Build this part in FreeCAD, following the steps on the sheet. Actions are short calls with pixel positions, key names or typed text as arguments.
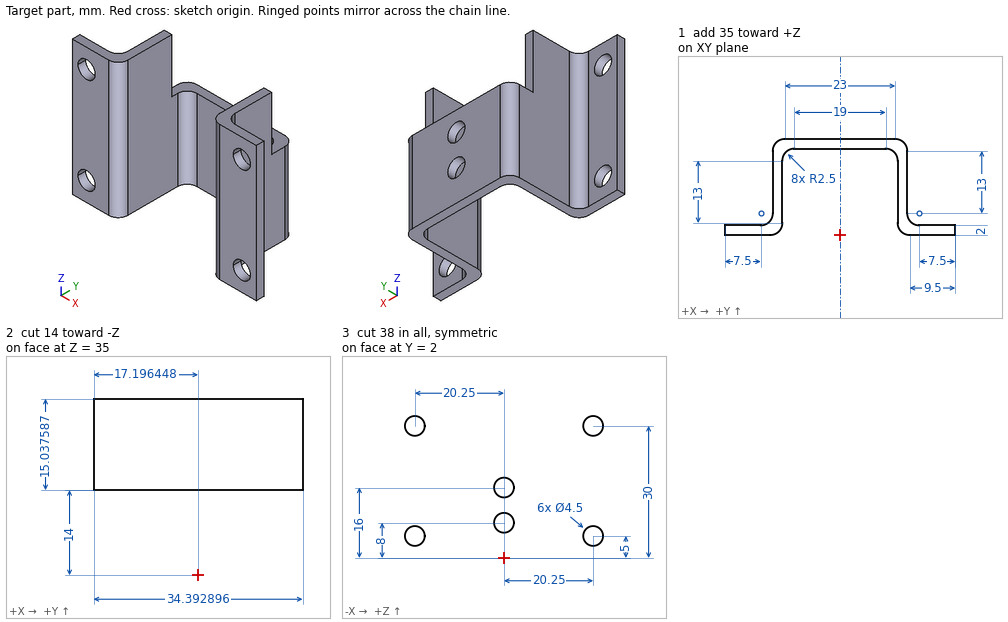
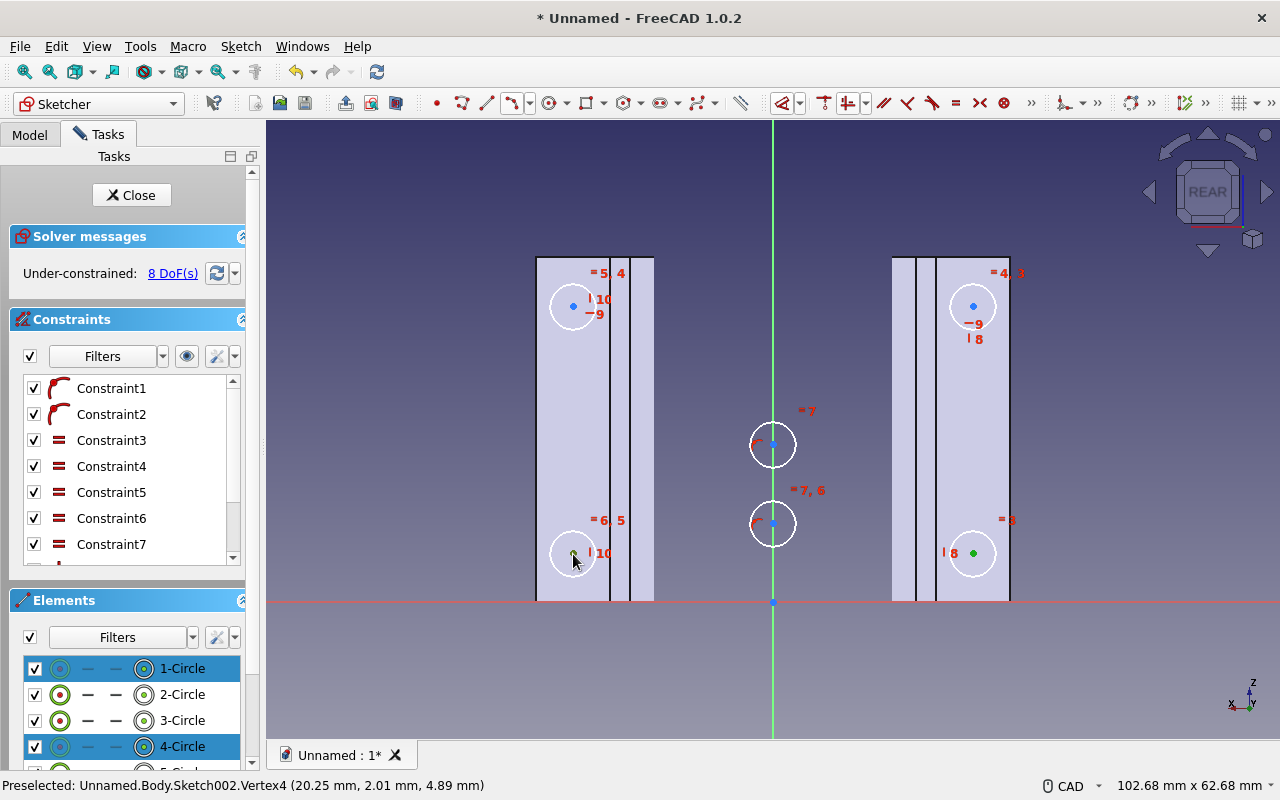
click(866, 104)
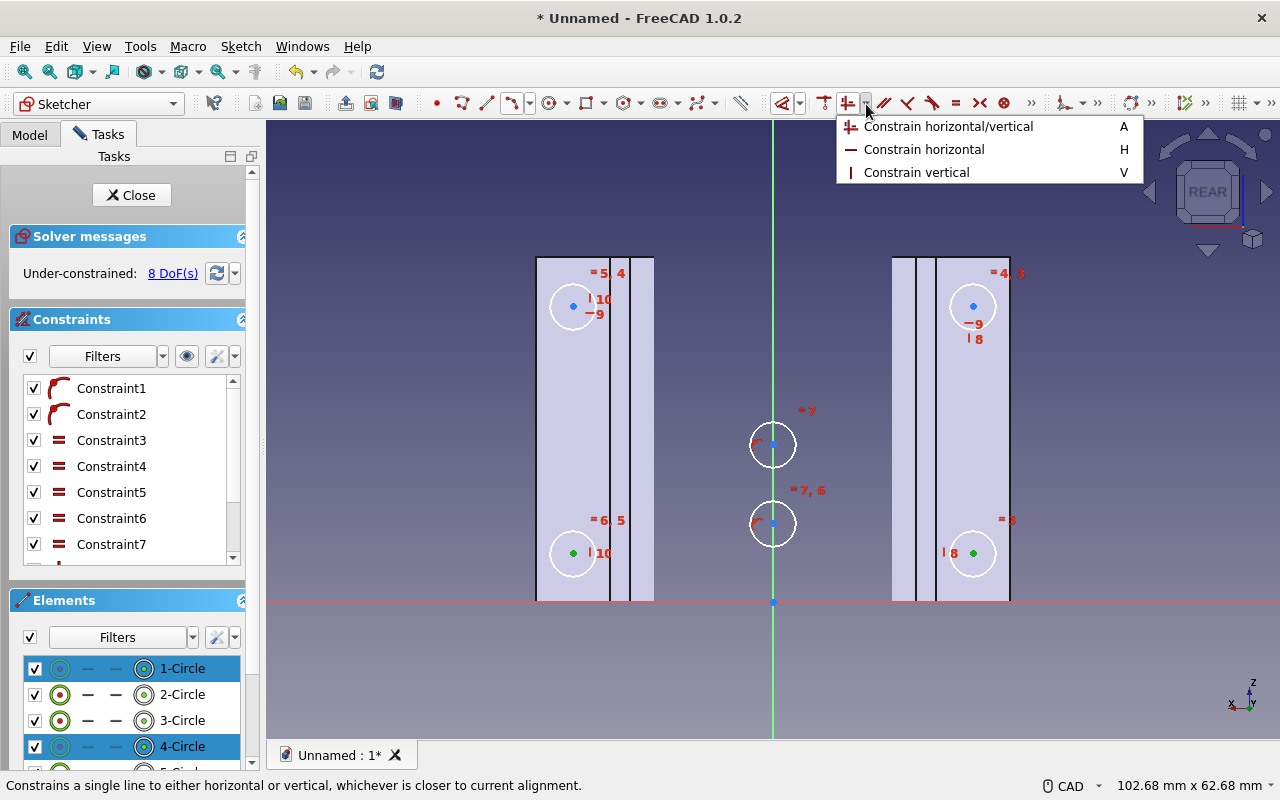
click(990, 150)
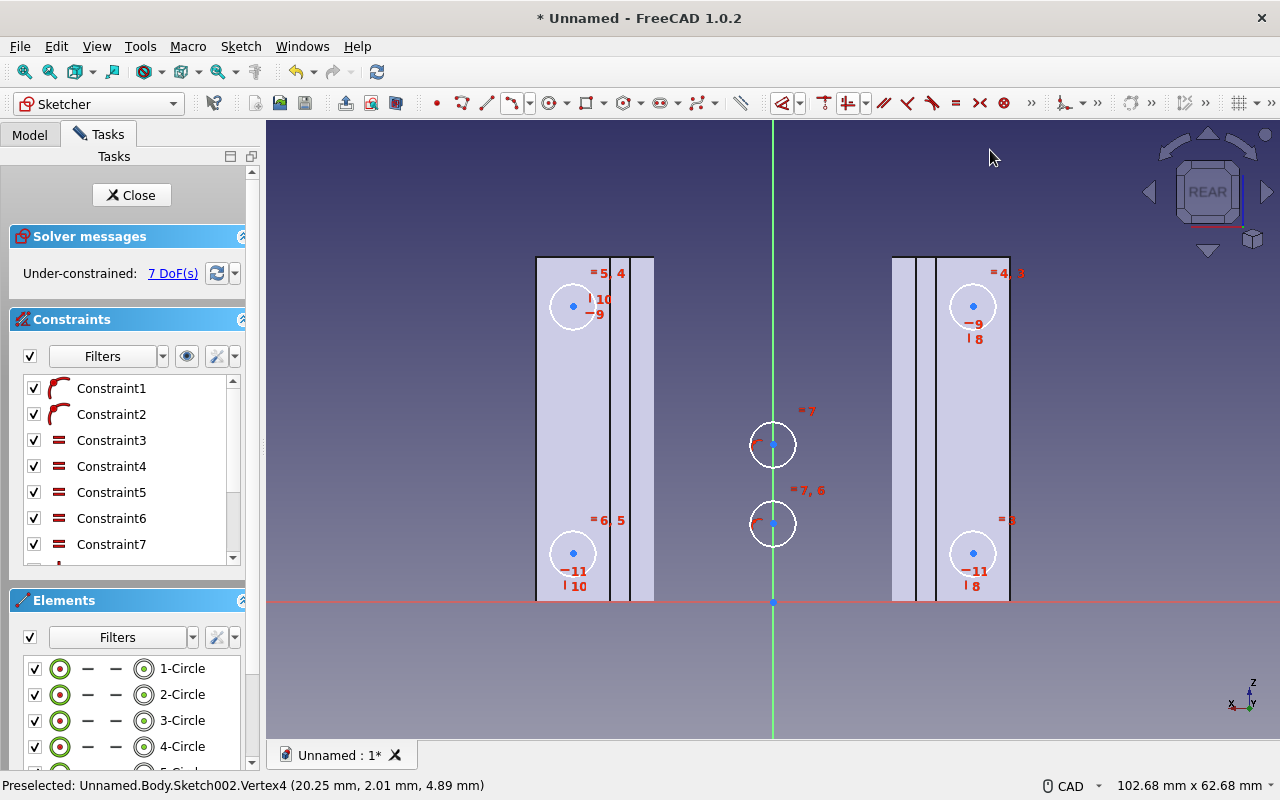
click(989, 538)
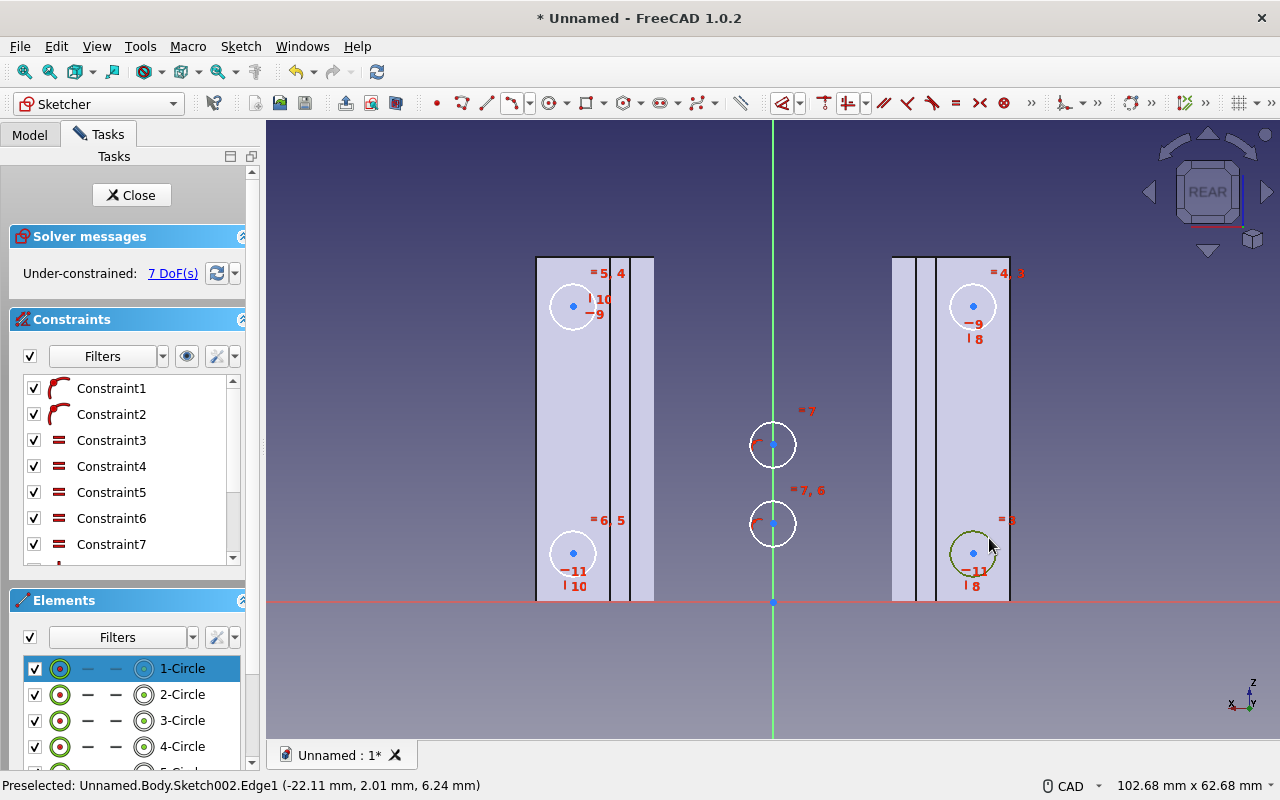
click(800, 104)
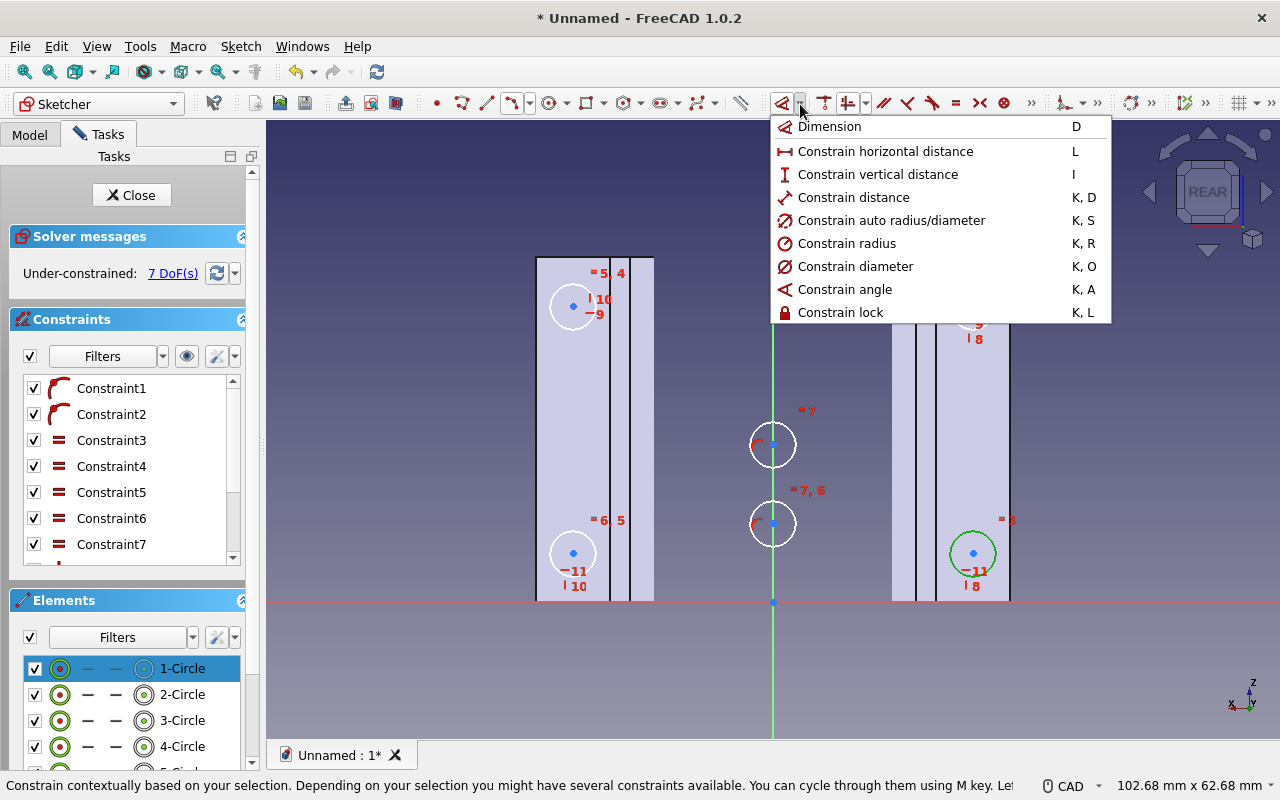
click(941, 266)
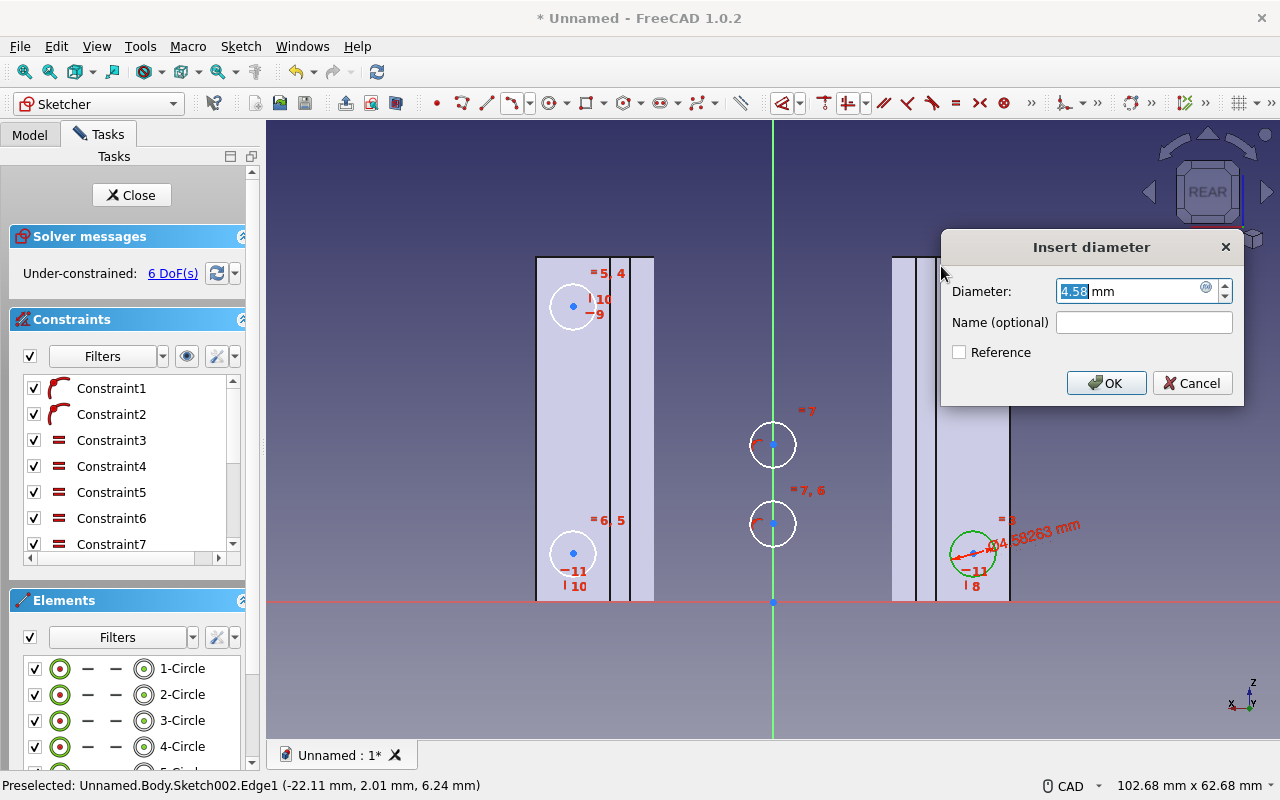
text(4.5)
key(Return)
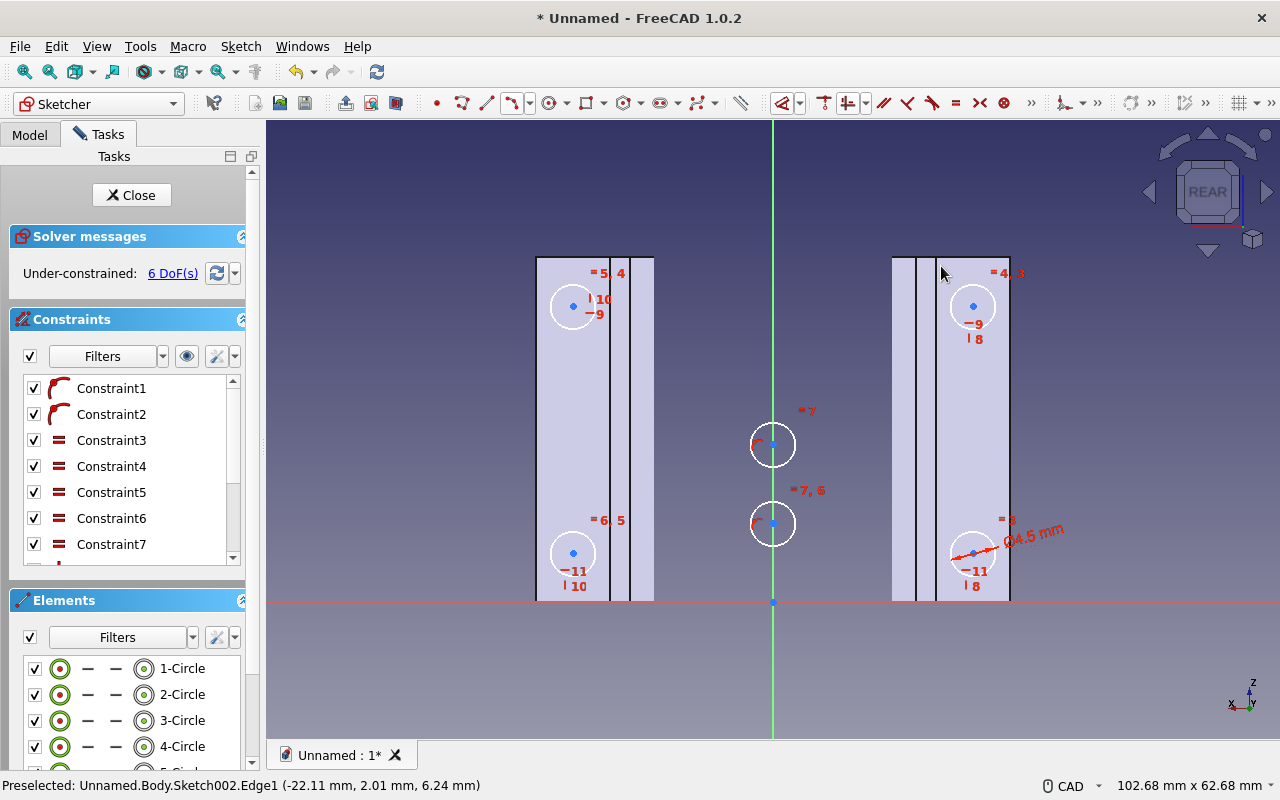
click(973, 554)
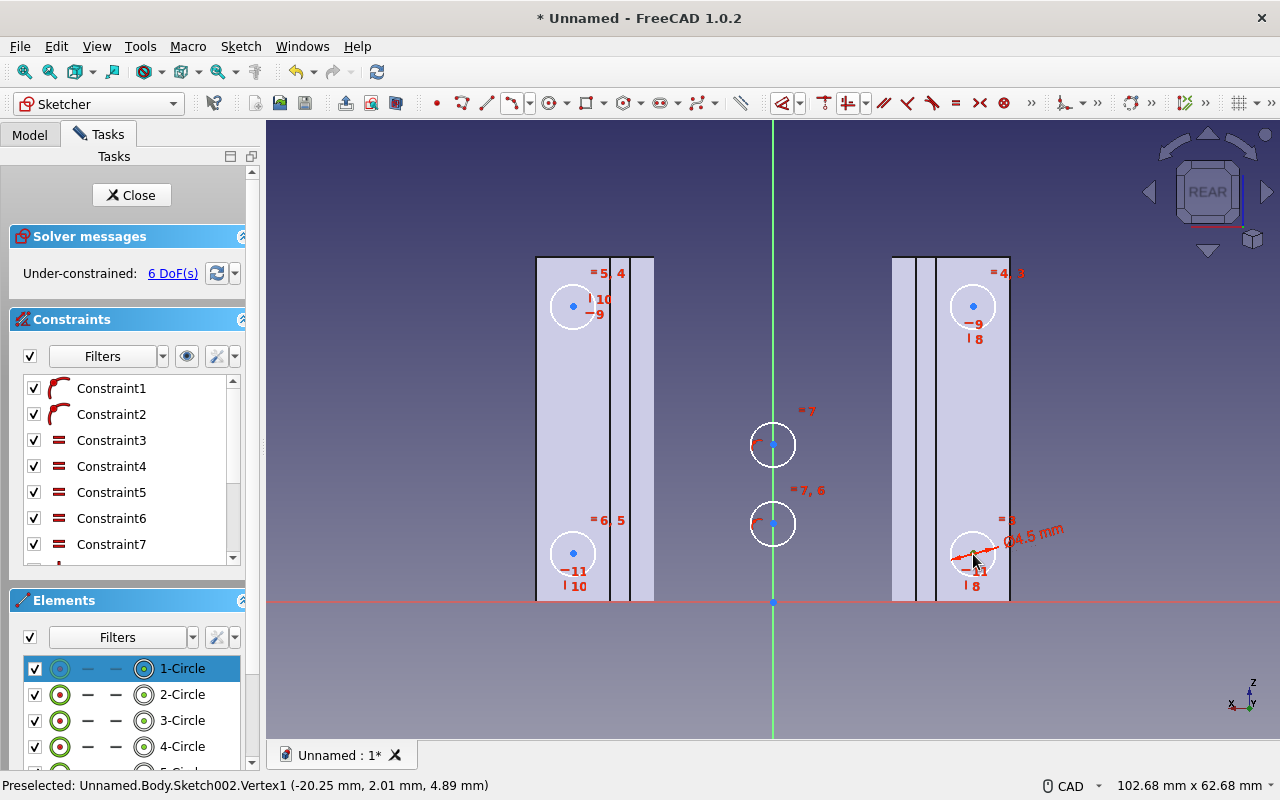
click(800, 104)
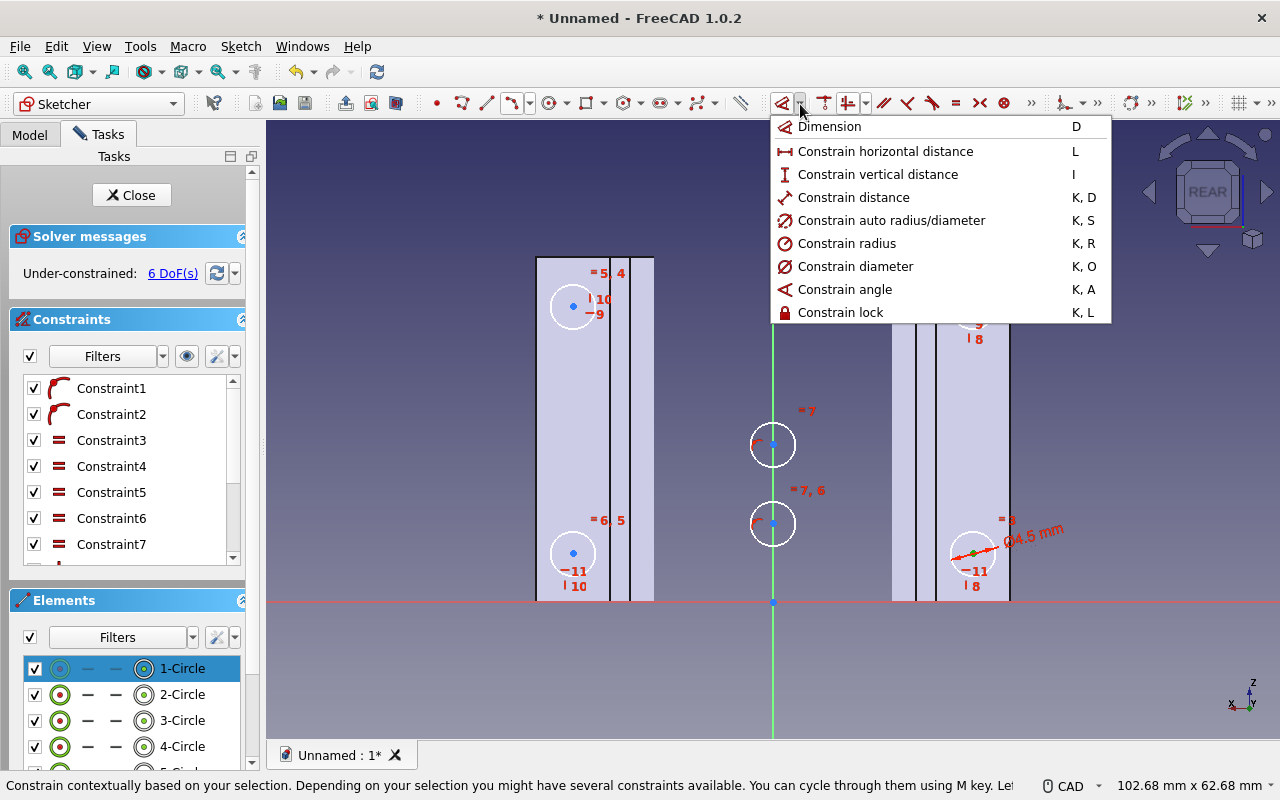
click(941, 174)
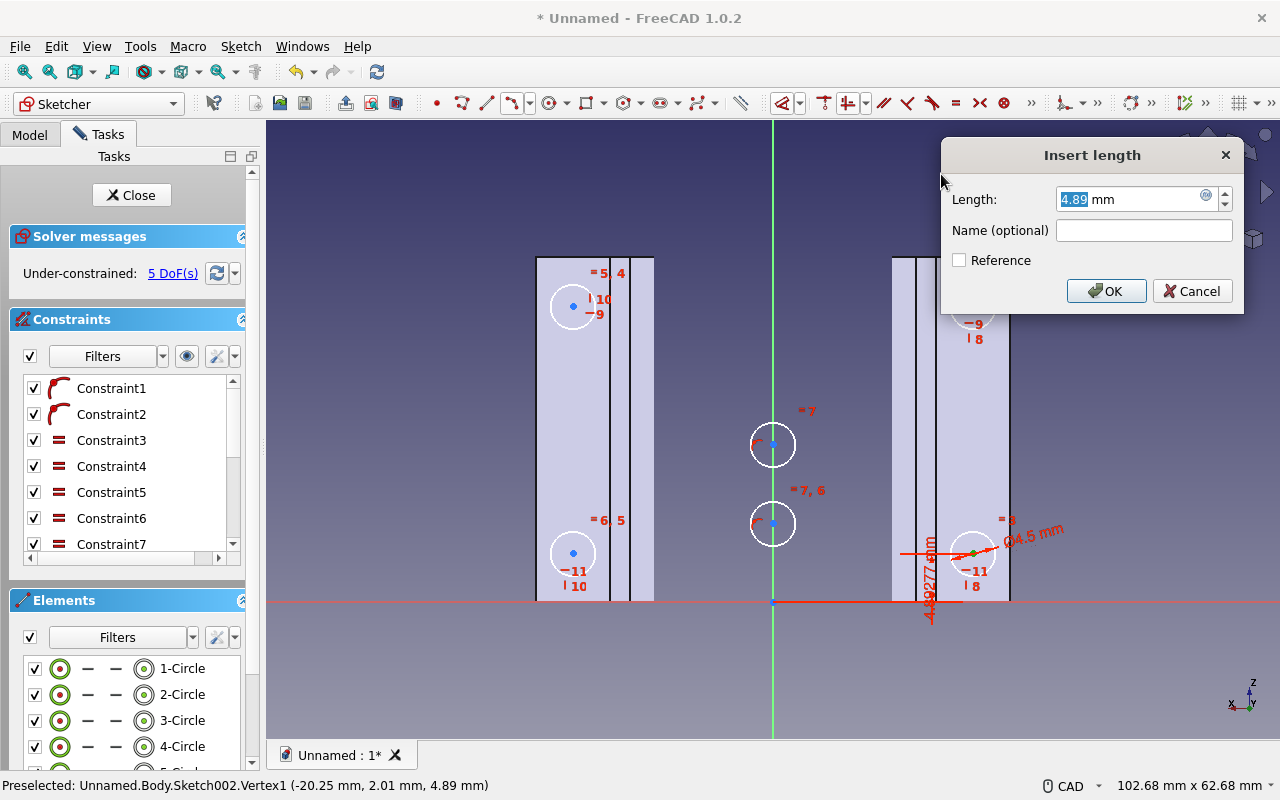
text(5)
key(Return)